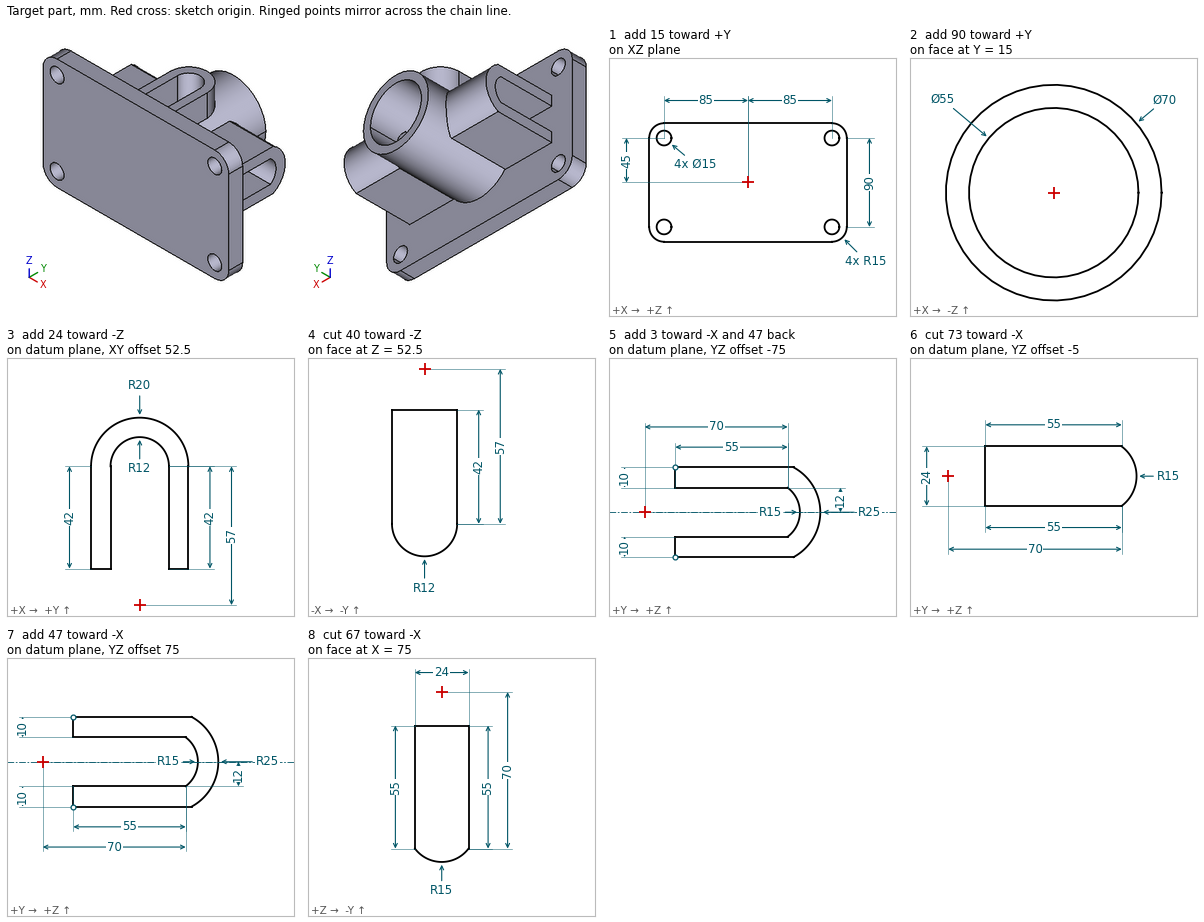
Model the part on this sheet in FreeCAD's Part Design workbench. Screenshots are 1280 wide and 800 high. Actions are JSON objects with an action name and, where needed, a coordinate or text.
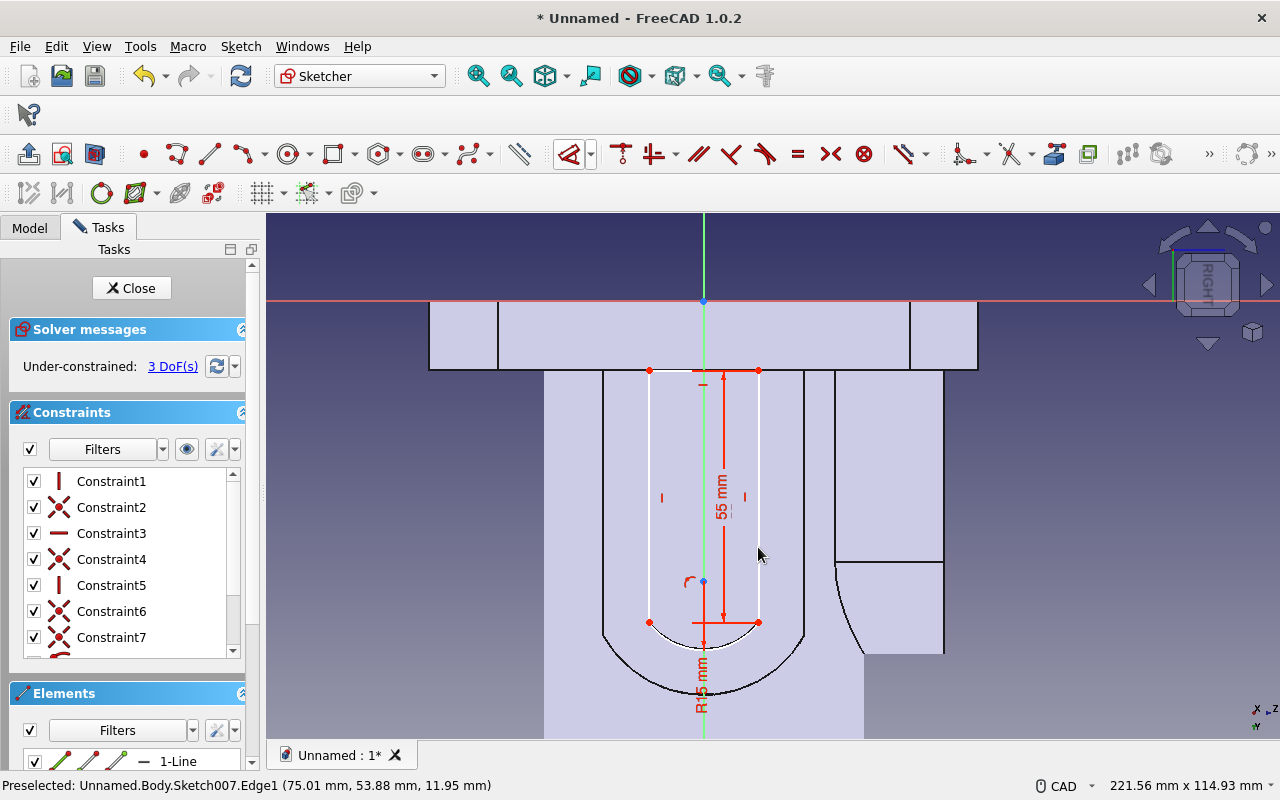
{"action": "left_click", "coordinate": [726, 371]}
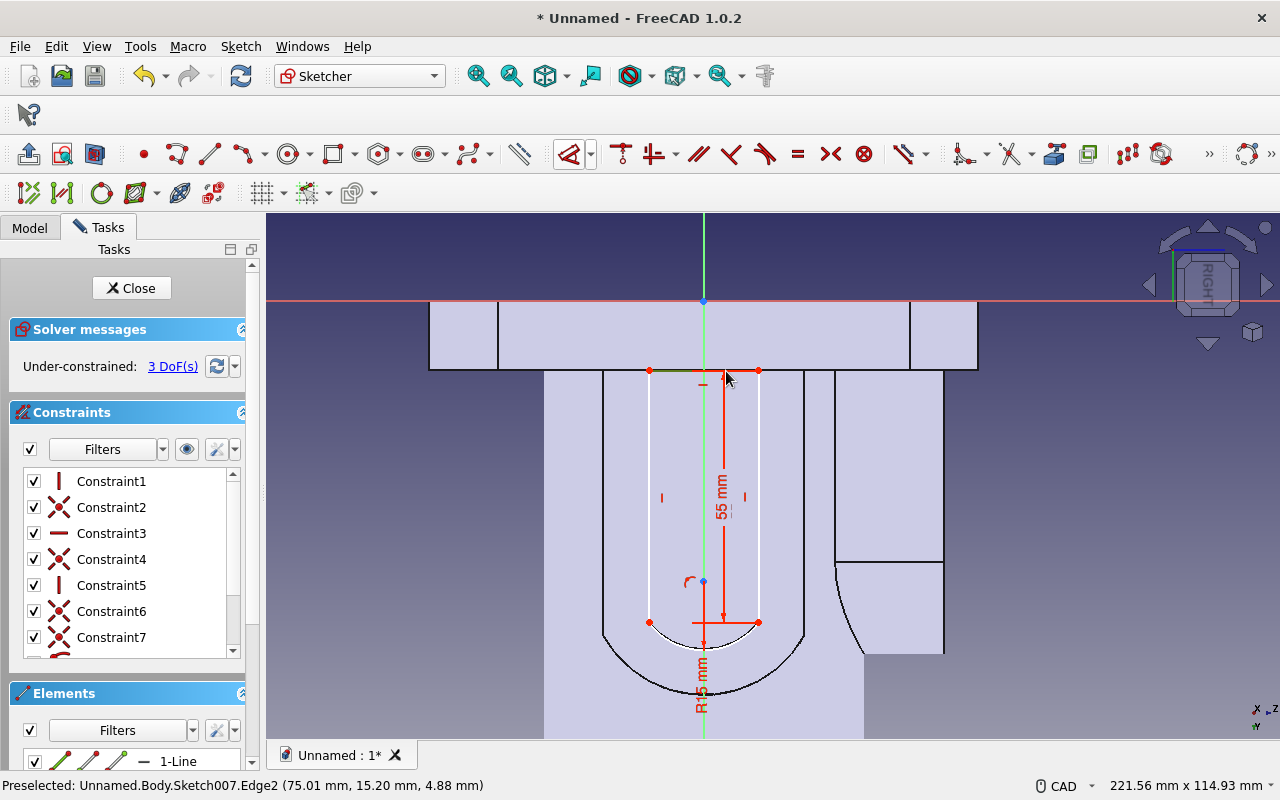
{"action": "left_click", "coordinate": [590, 154]}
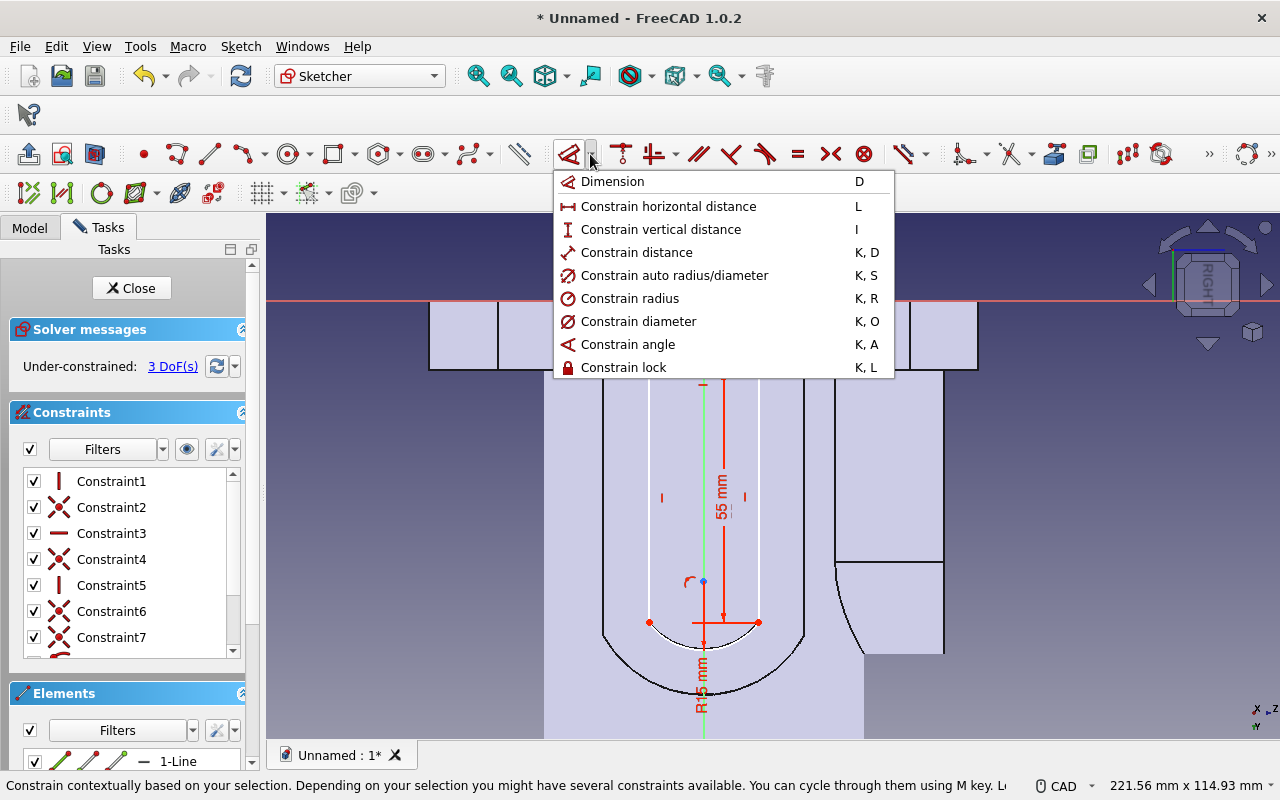
{"action": "left_click", "coordinate": [724, 206]}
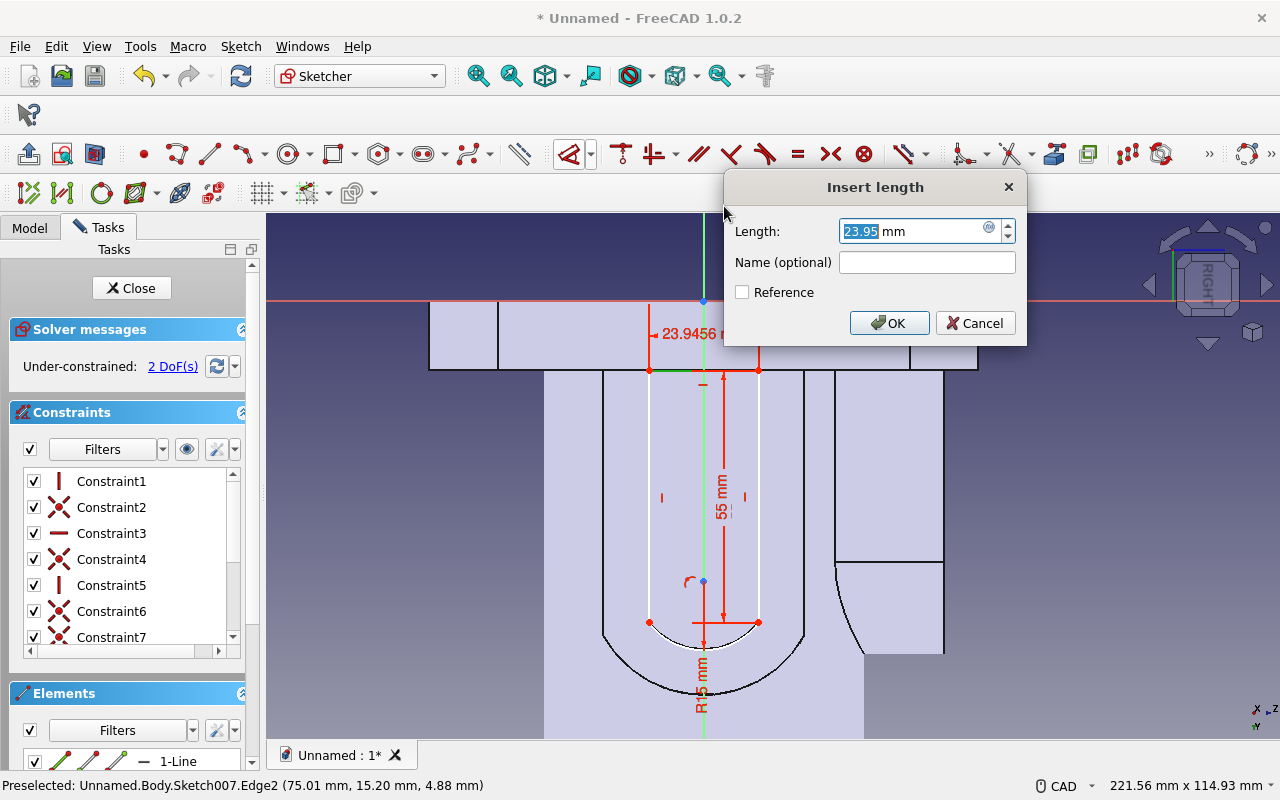
{"action": "type", "text": "24"}
{"action": "key", "text": "Return"}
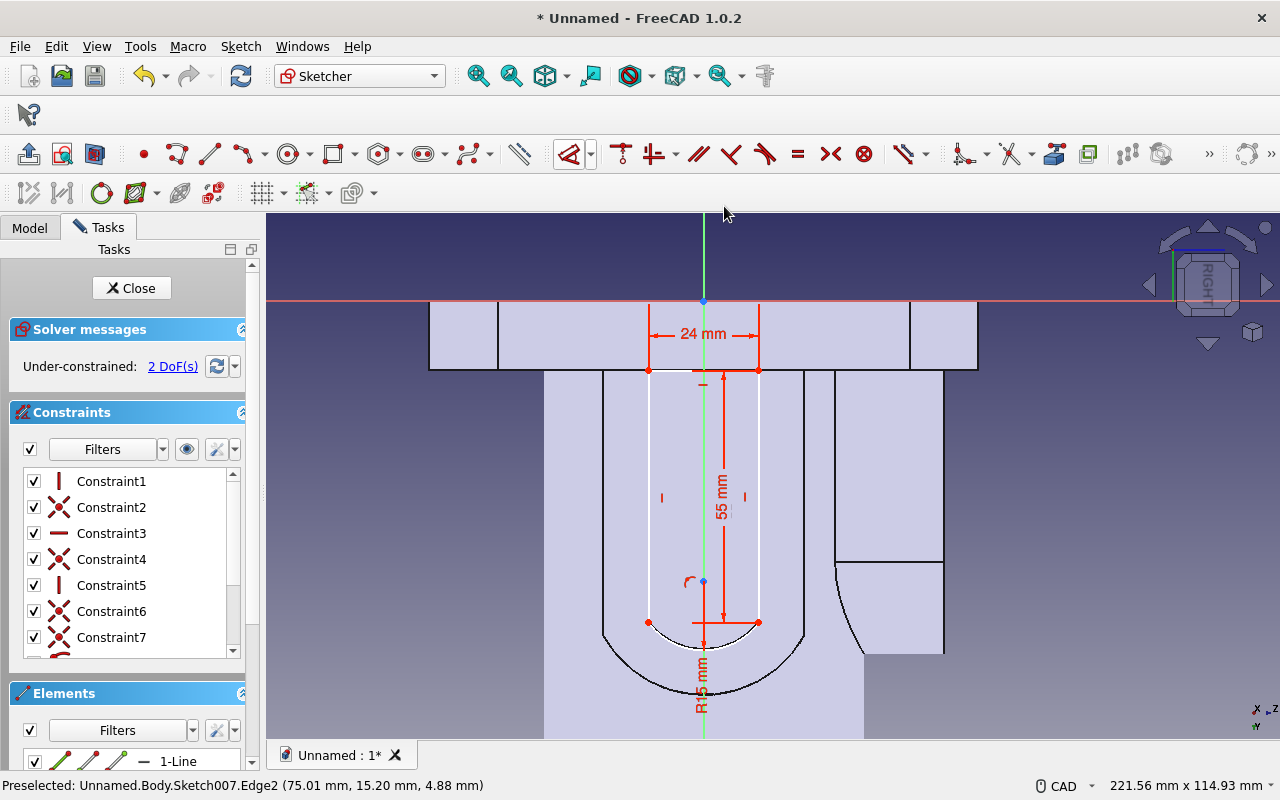
{"action": "left_click", "coordinate": [649, 447]}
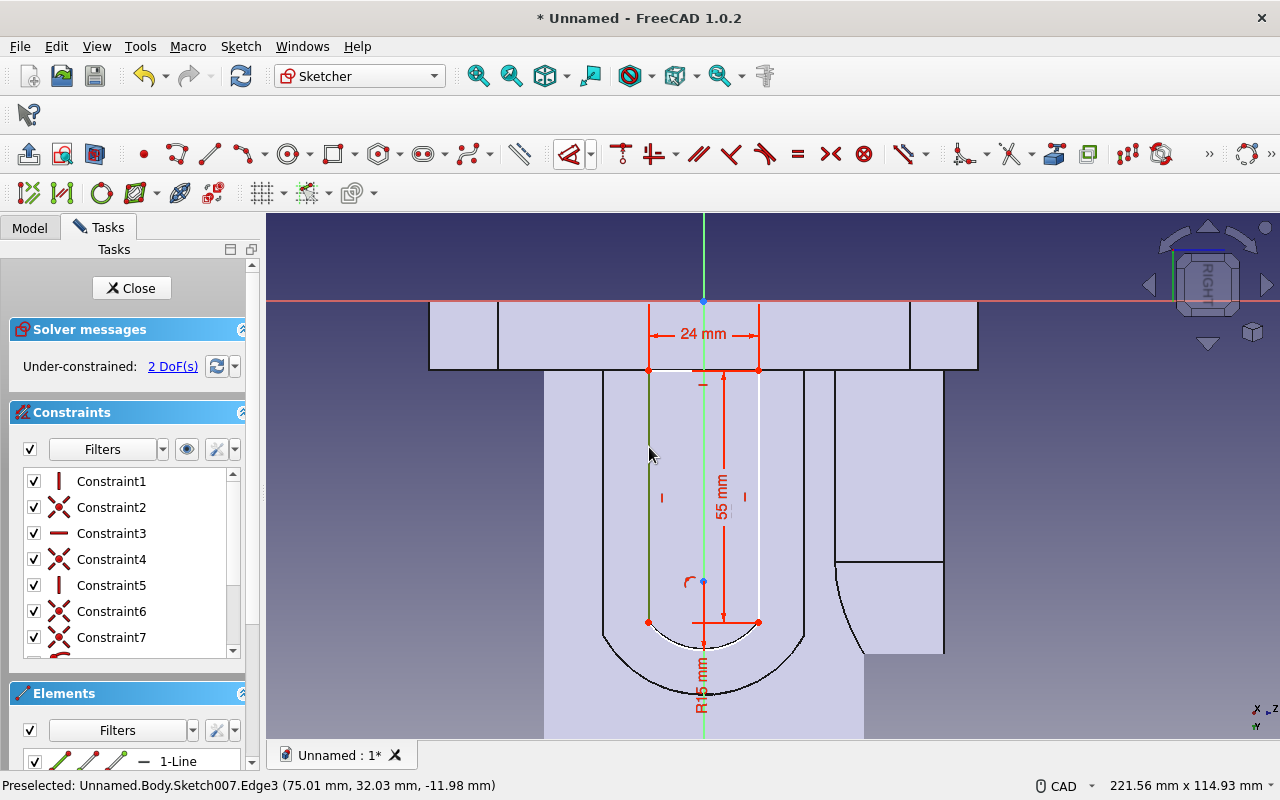
{"action": "key", "text": "i"}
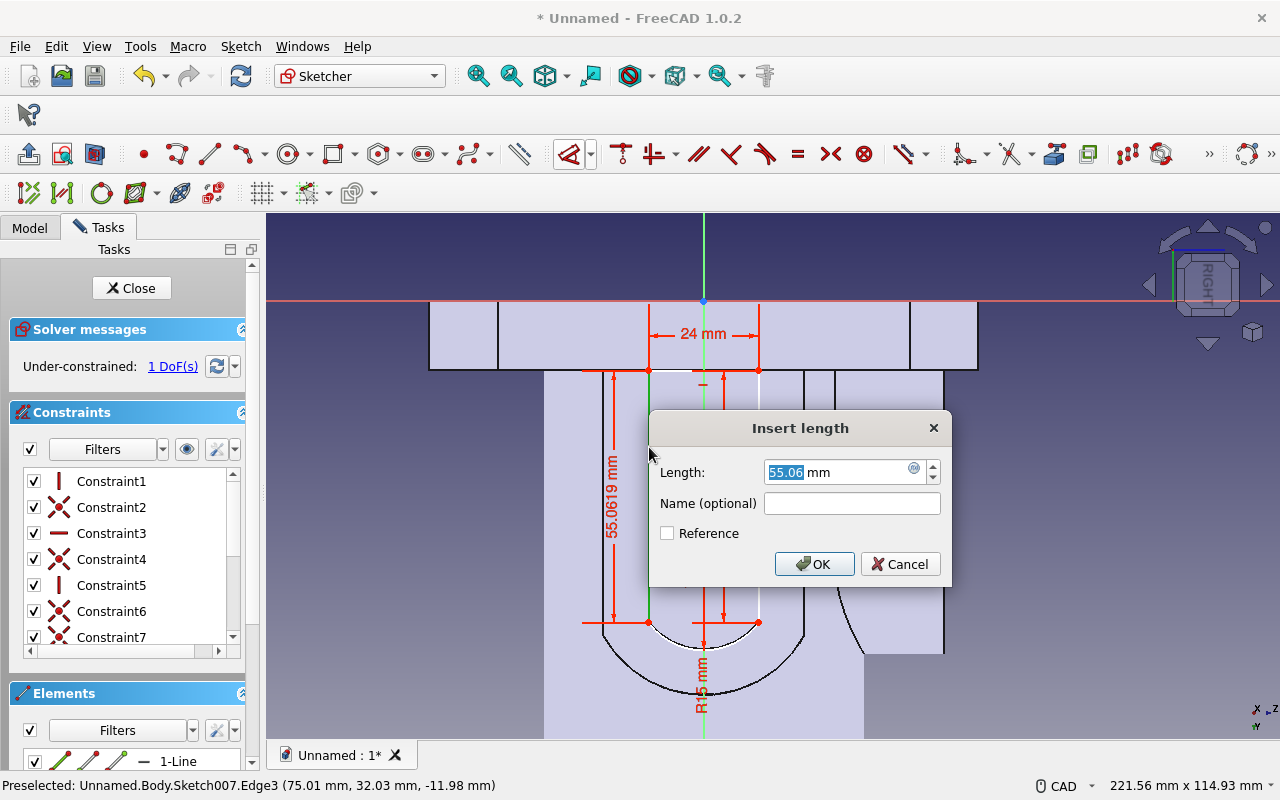
{"action": "type", "text": "55"}
{"action": "key", "text": "Return"}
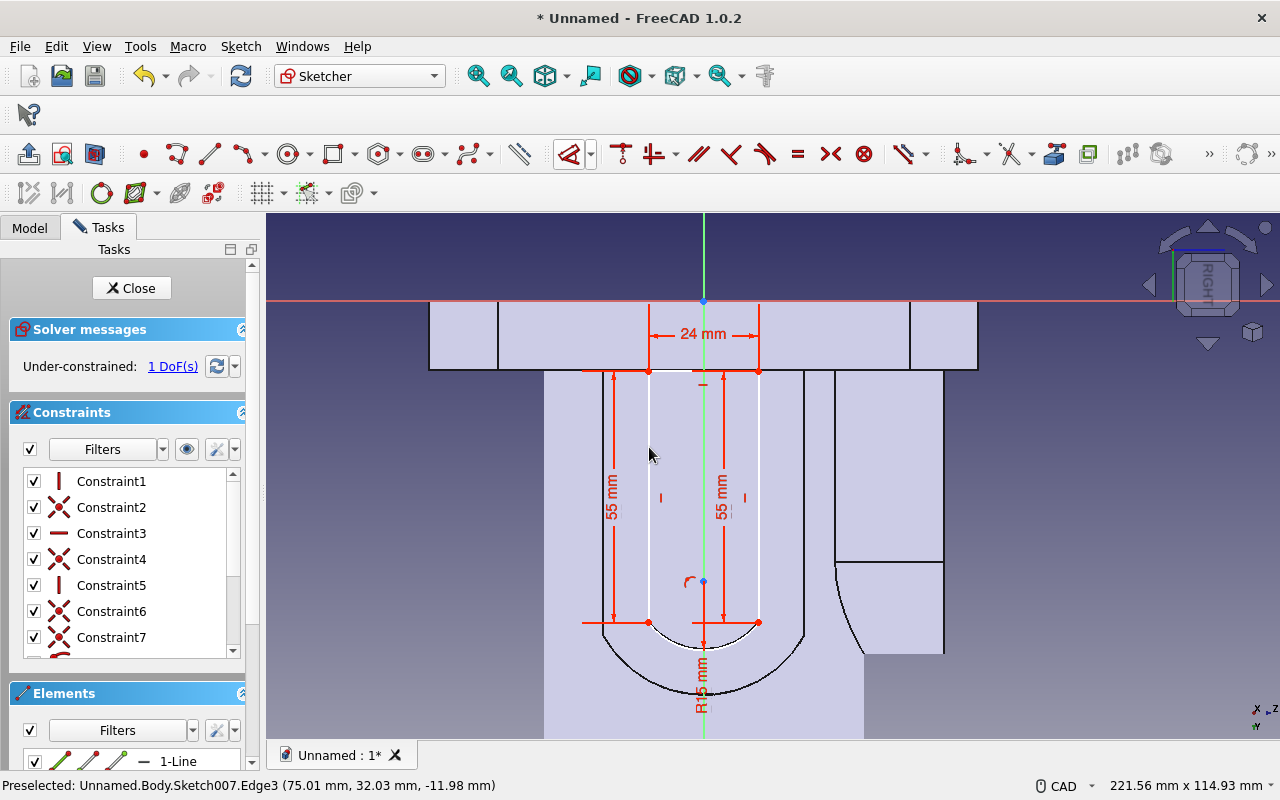
{"action": "left_click", "coordinate": [759, 623]}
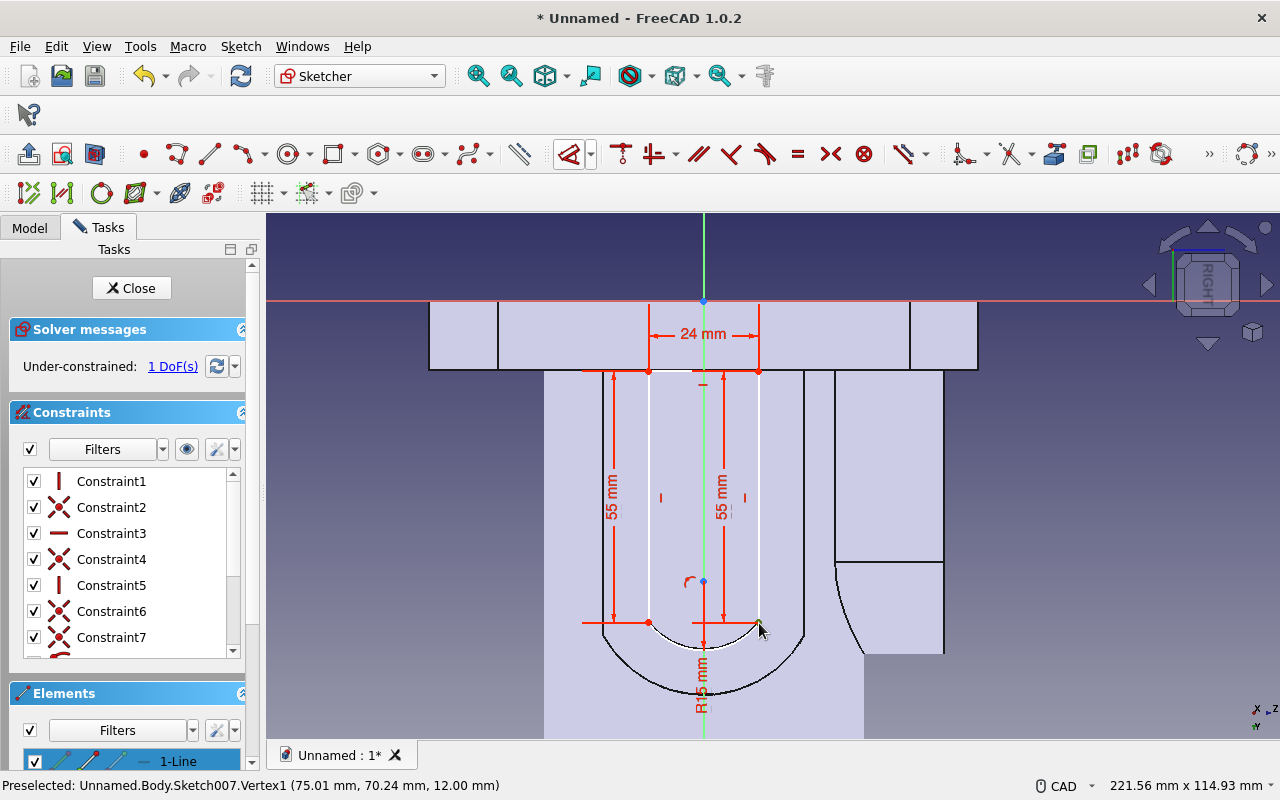
{"action": "key", "text": "i"}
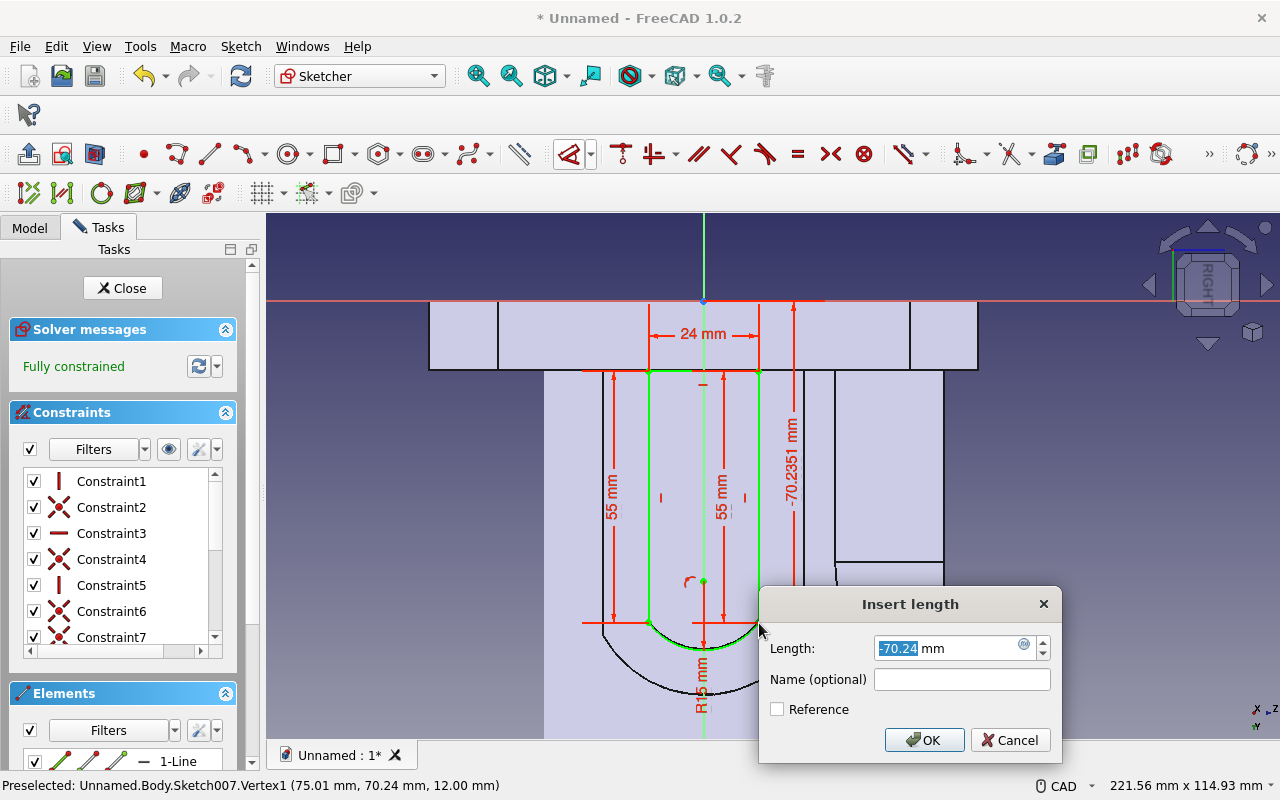
{"action": "type", "text": "-70"}
{"action": "key", "text": "Return"}